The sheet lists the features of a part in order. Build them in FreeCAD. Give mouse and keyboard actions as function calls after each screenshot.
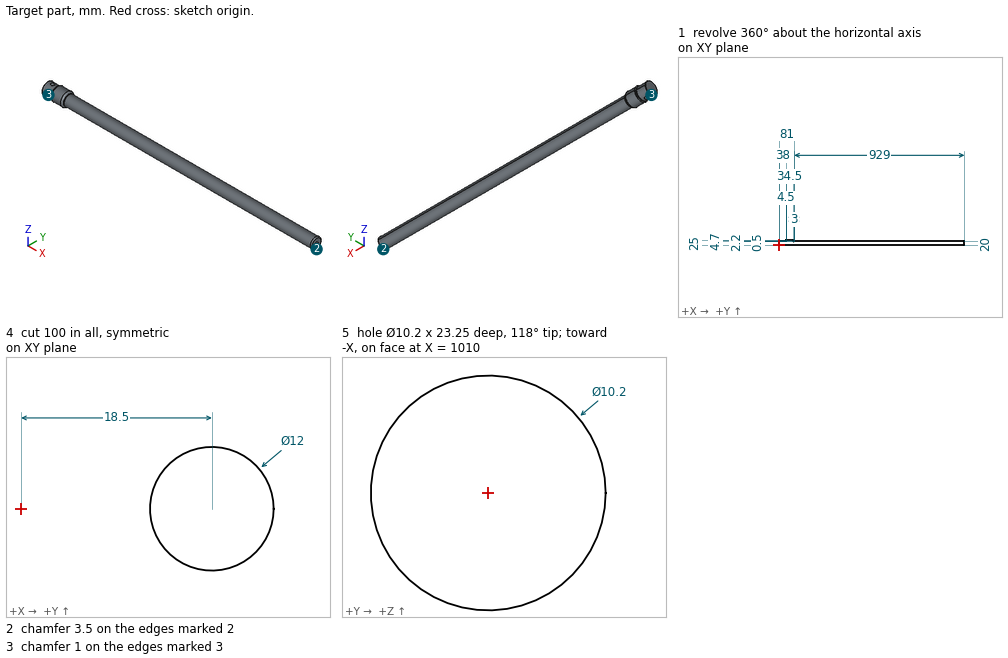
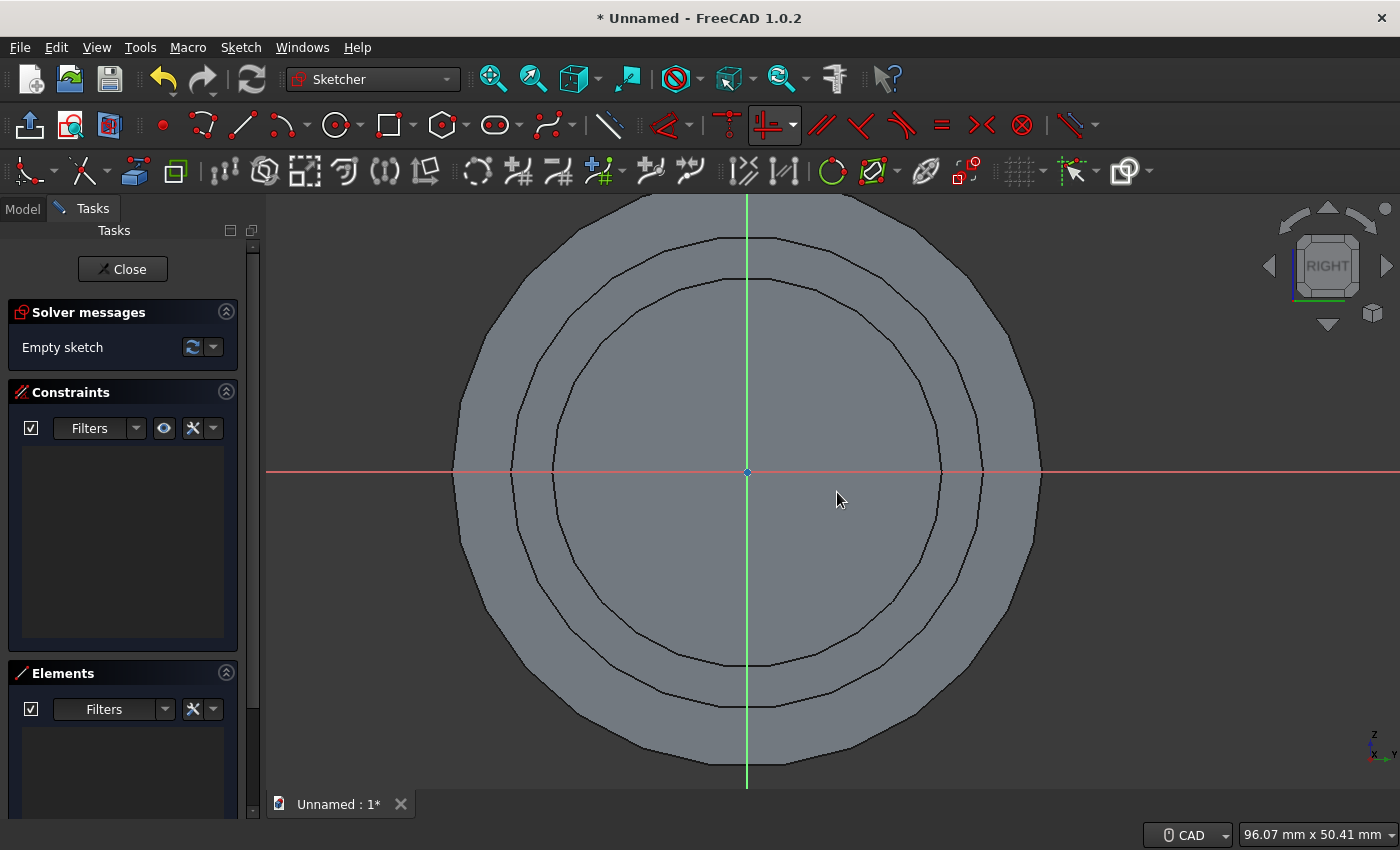
scroll(740, 464, up, 6)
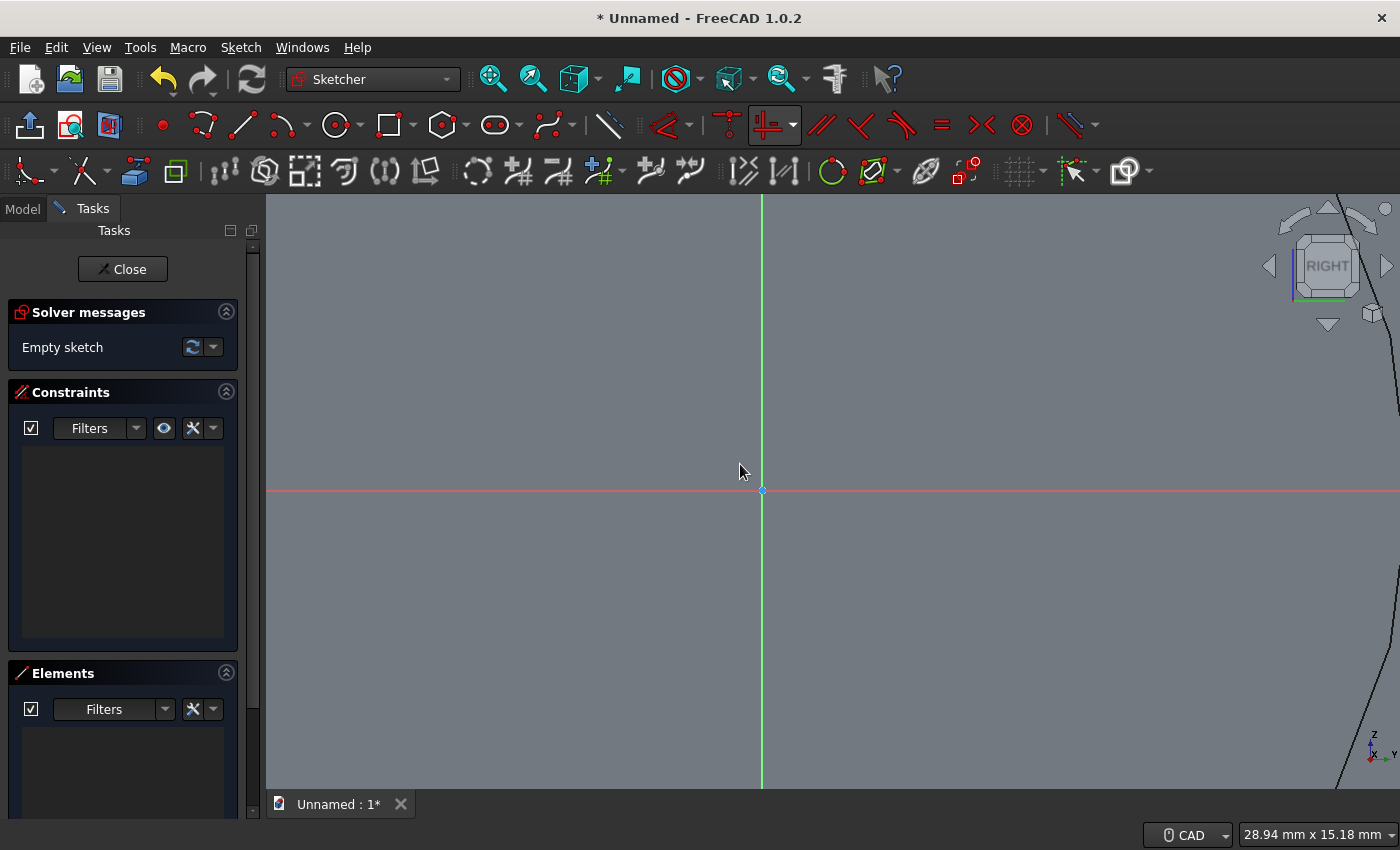
click(336, 126)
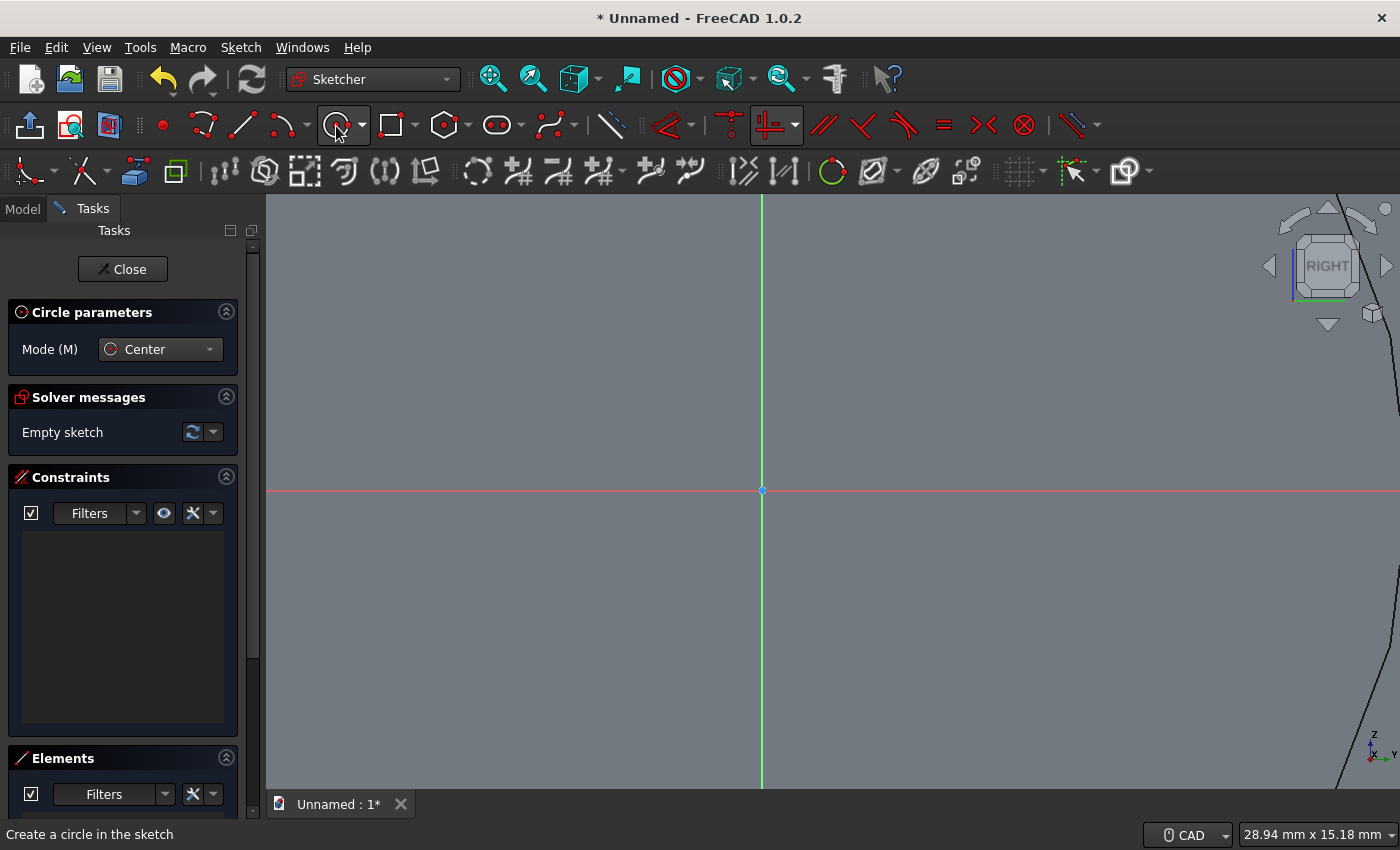
click(762, 491)
click(904, 349)
key(Escape)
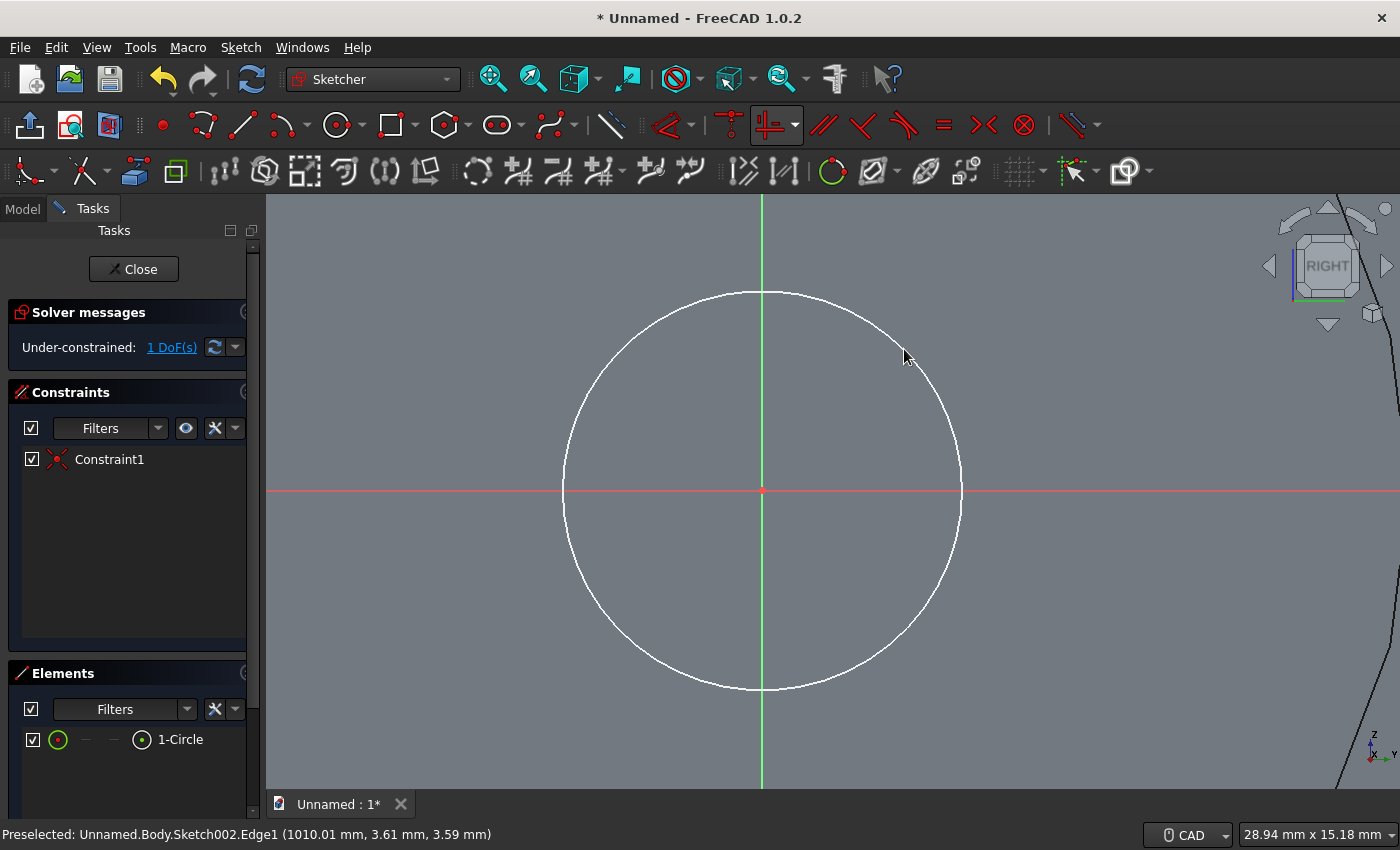
click(666, 126)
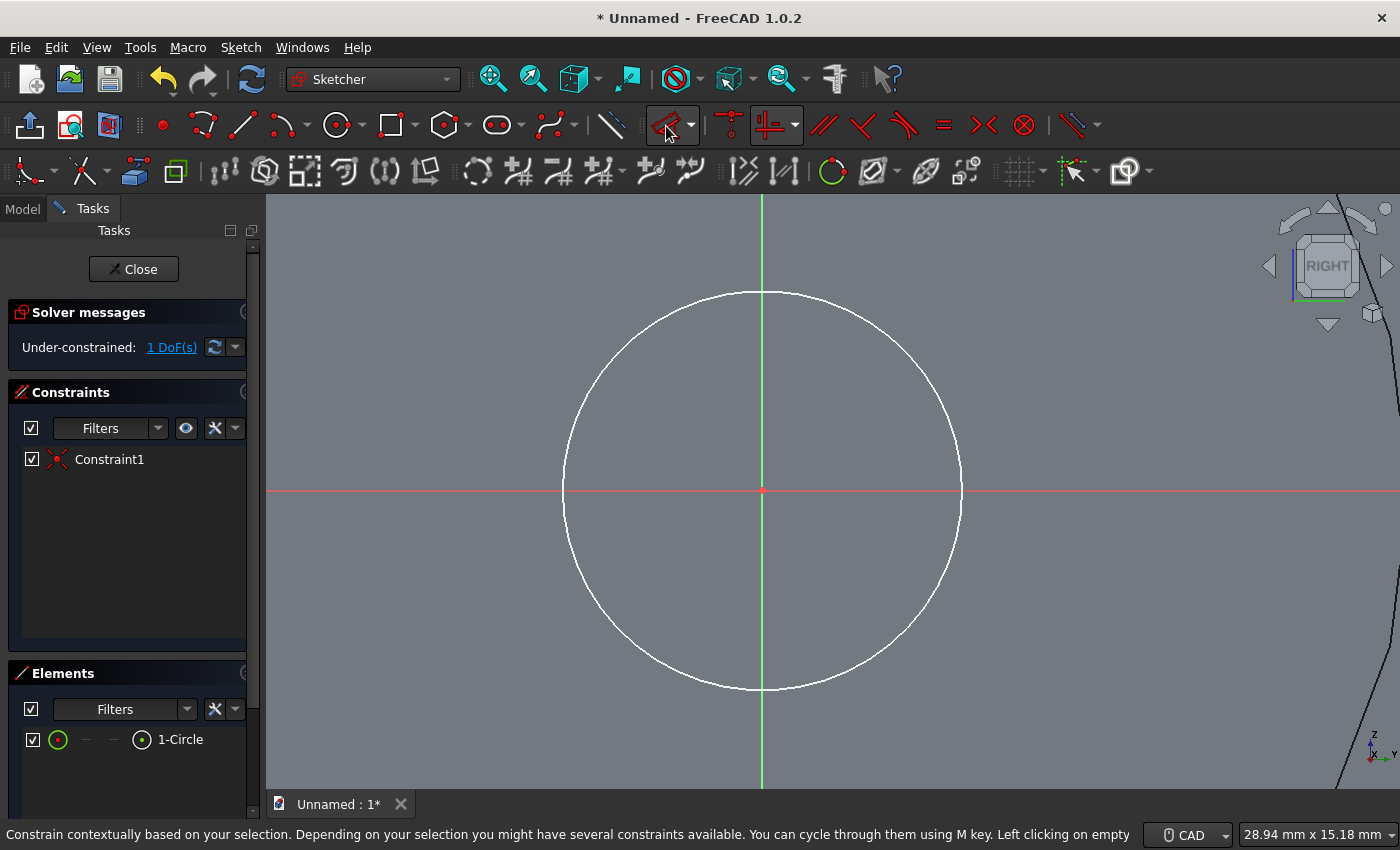
click(903, 349)
click(926, 326)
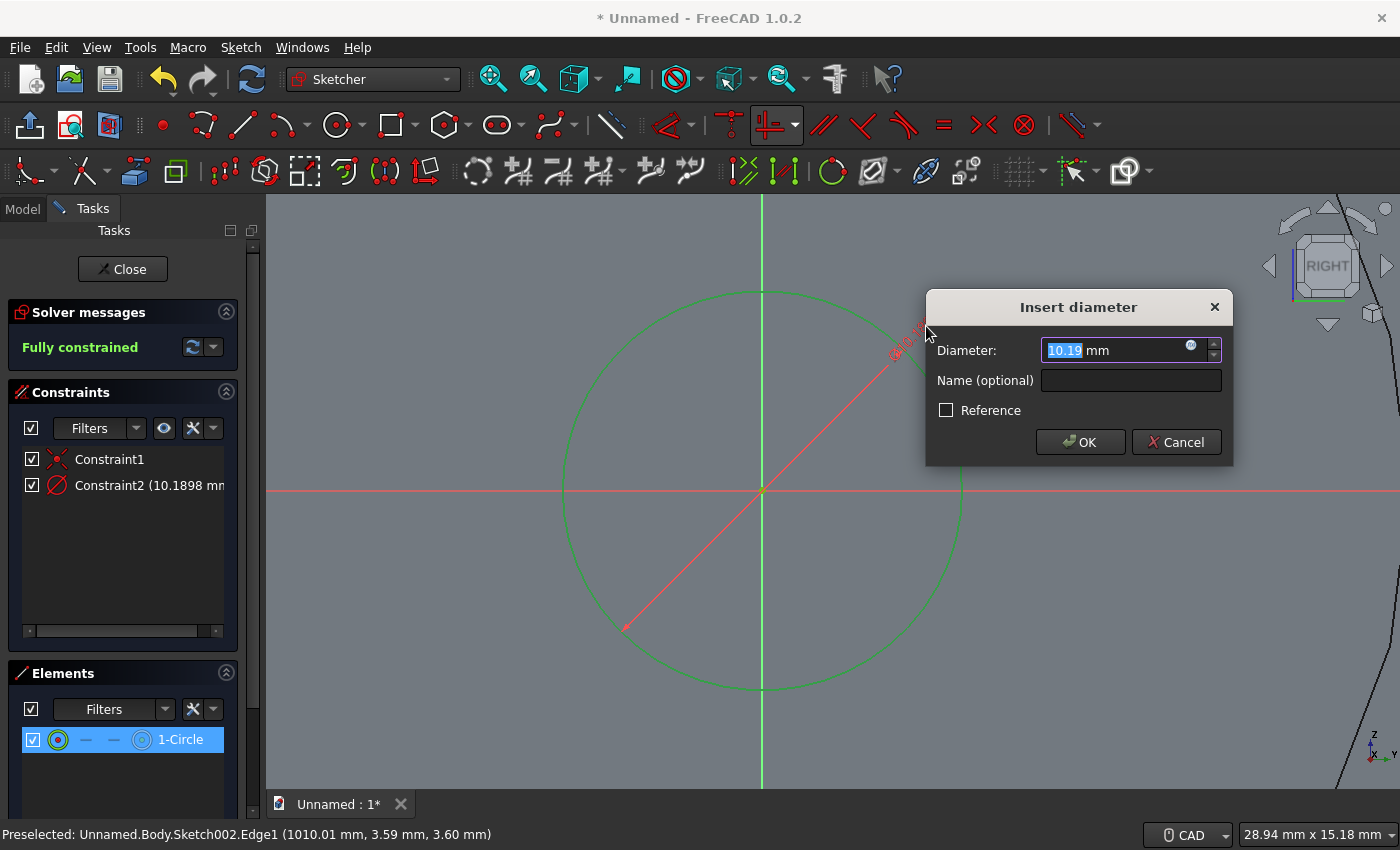
text(10.2)
key(Return)
key(Escape)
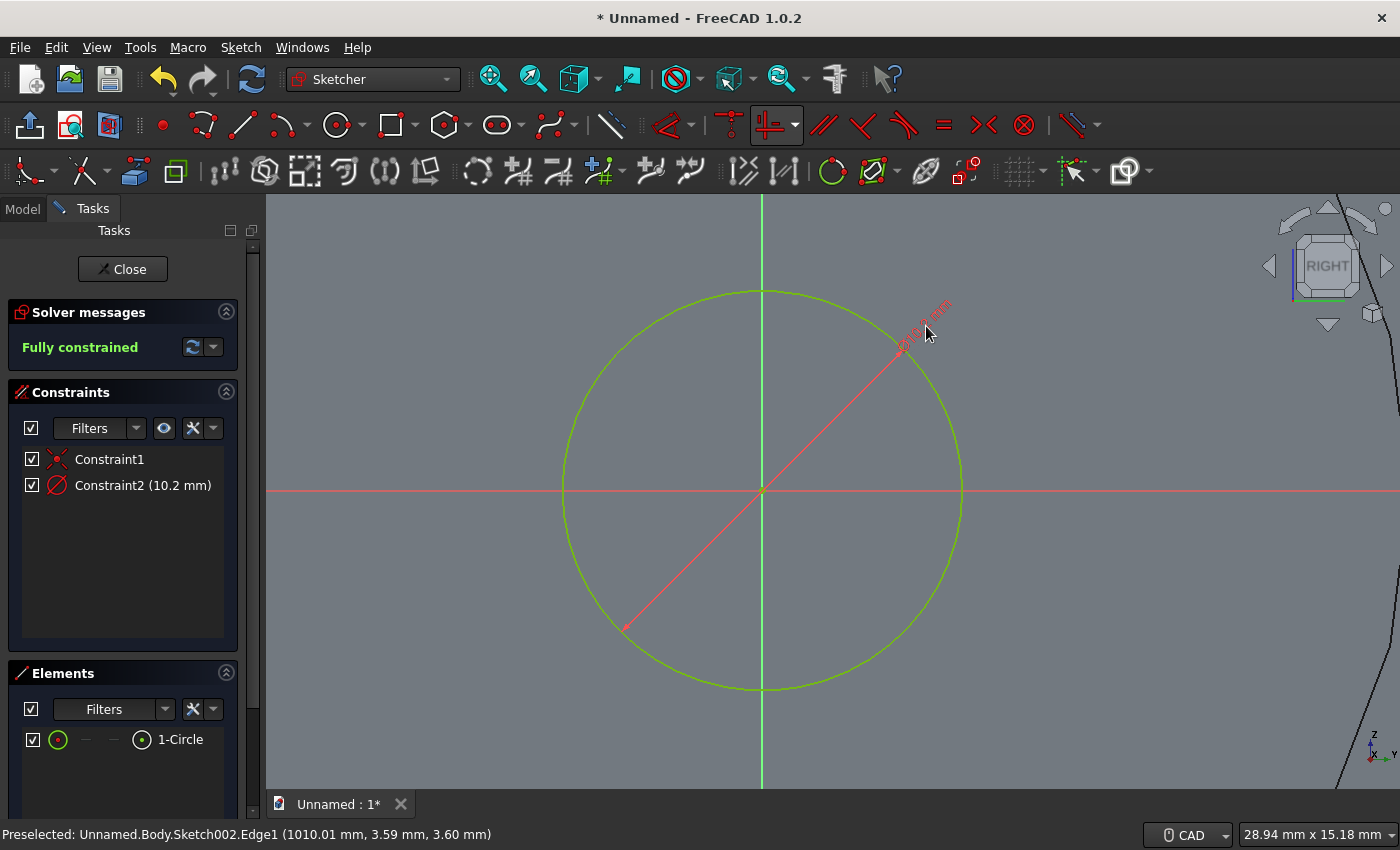
click(123, 269)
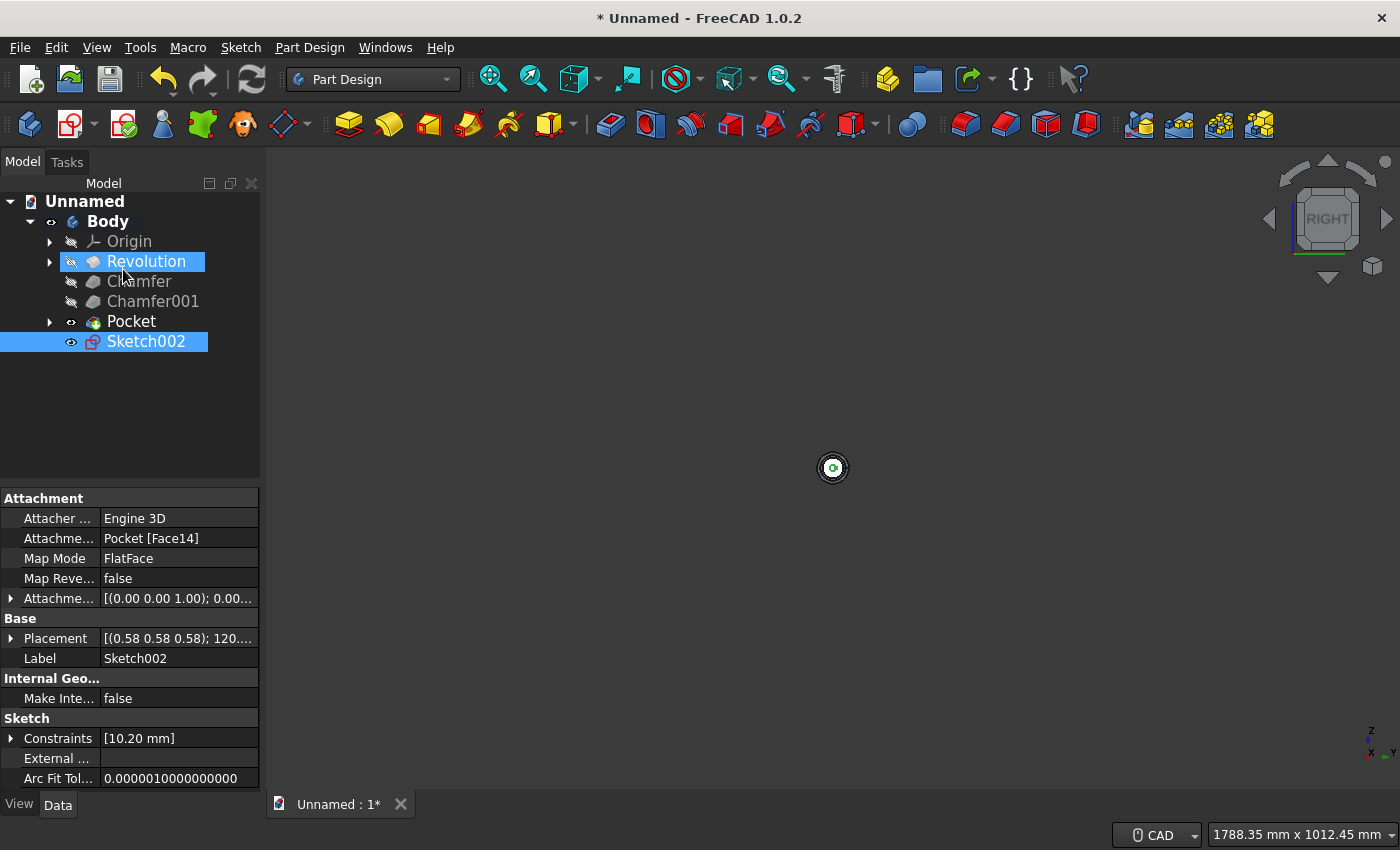
click(652, 124)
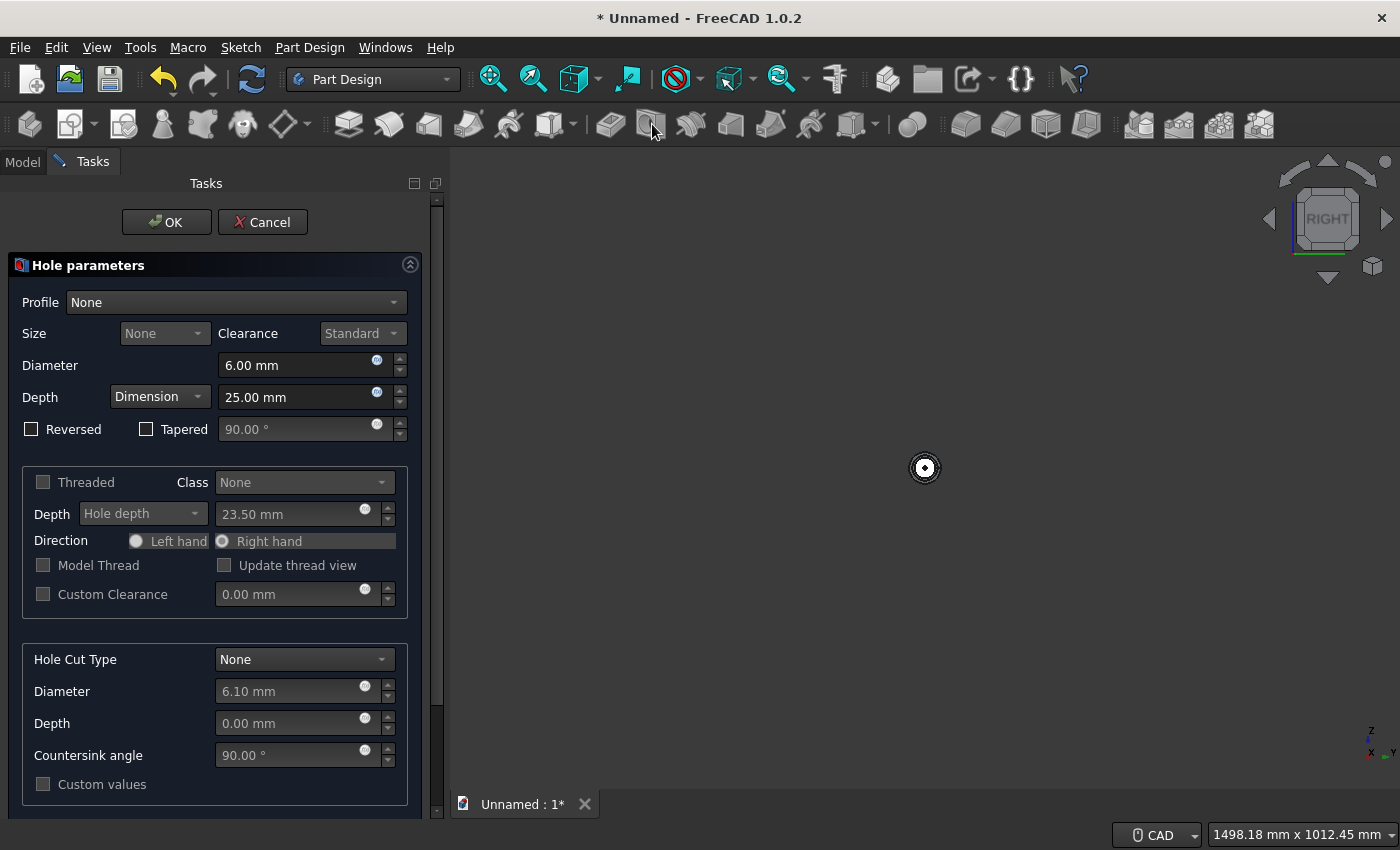
triple_click(305, 365)